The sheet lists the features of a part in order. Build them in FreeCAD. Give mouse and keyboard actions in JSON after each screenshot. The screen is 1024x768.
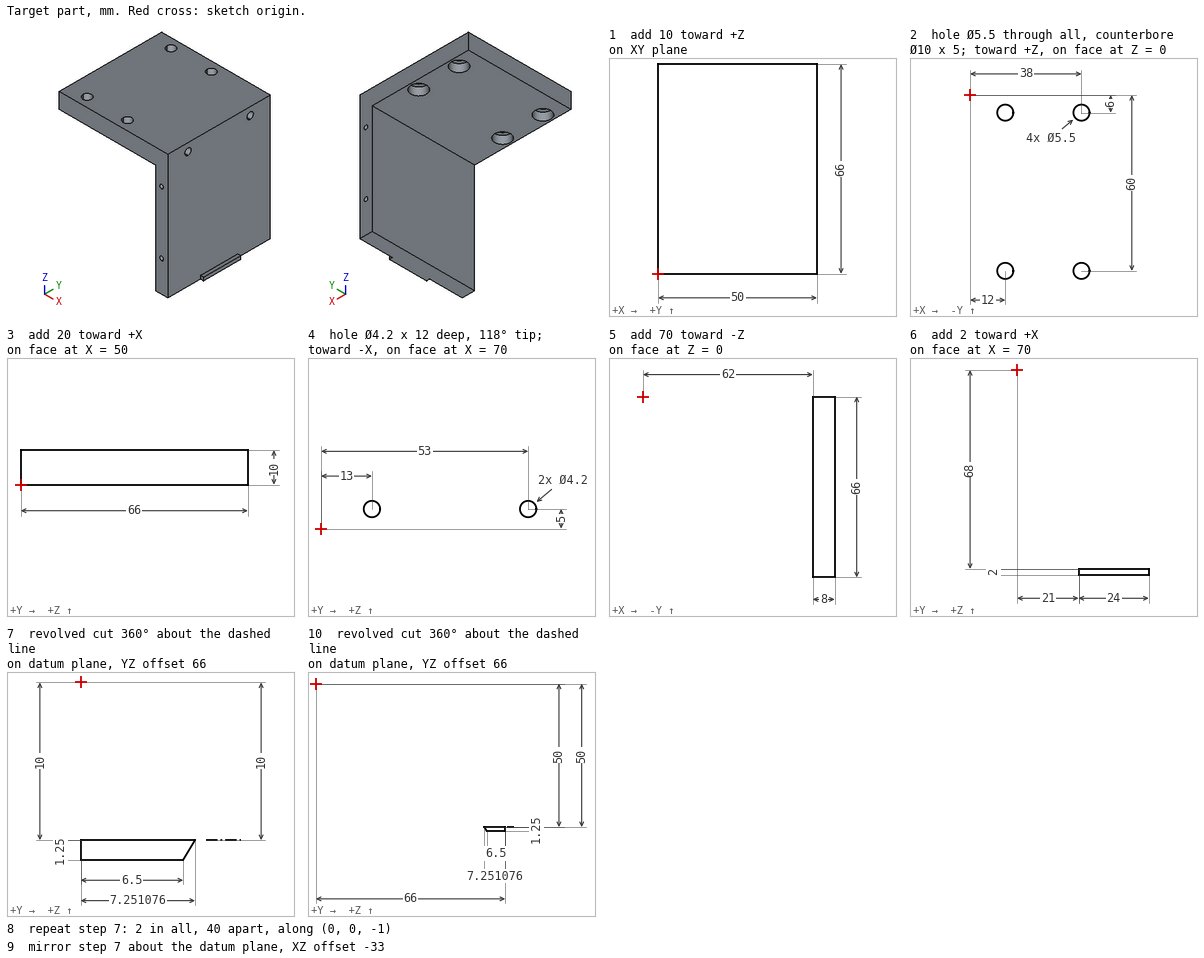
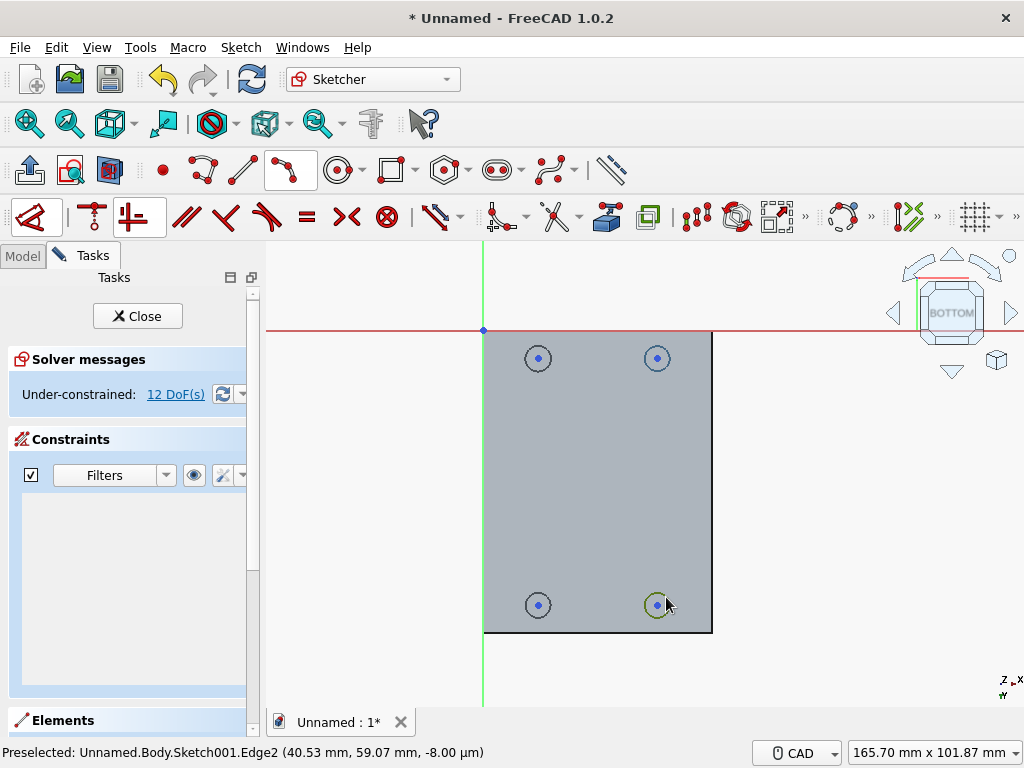
{"action": "left_click", "coordinate": [547, 597]}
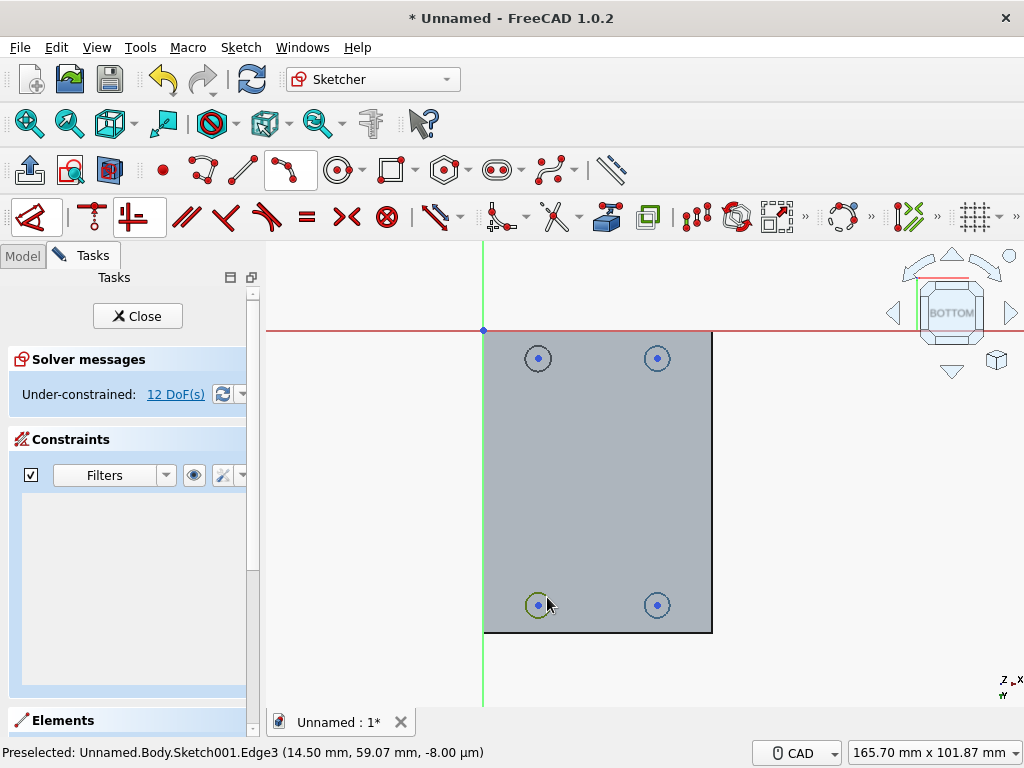
{"action": "left_click", "coordinate": [547, 350]}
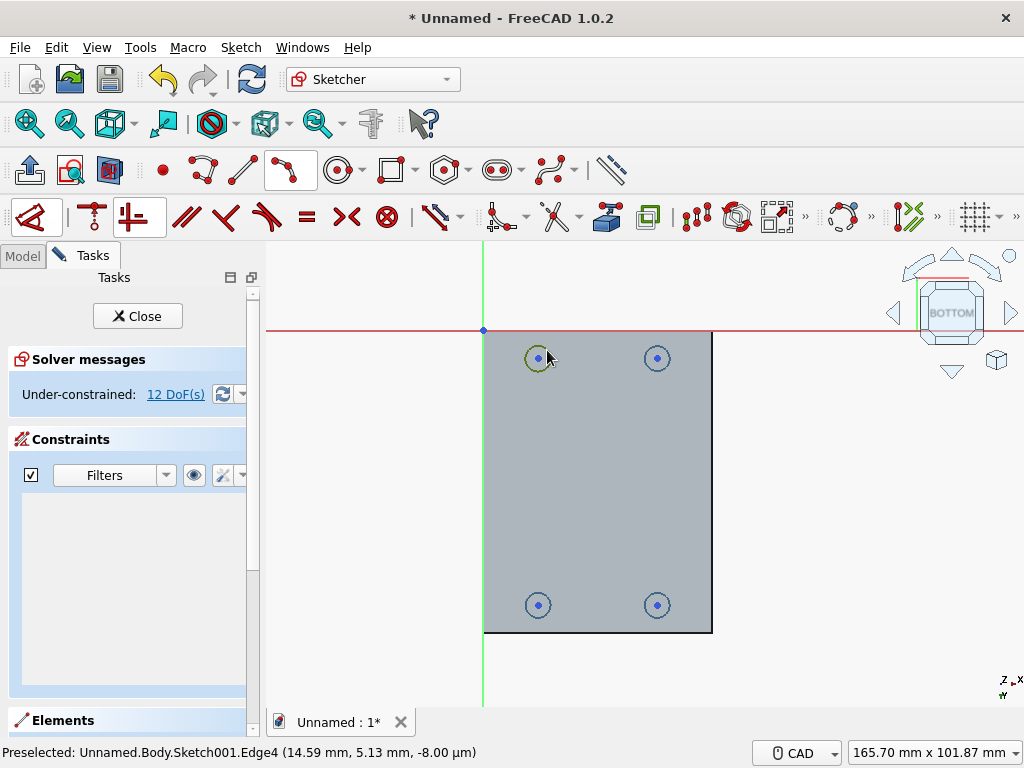
{"action": "left_click", "coordinate": [308, 218]}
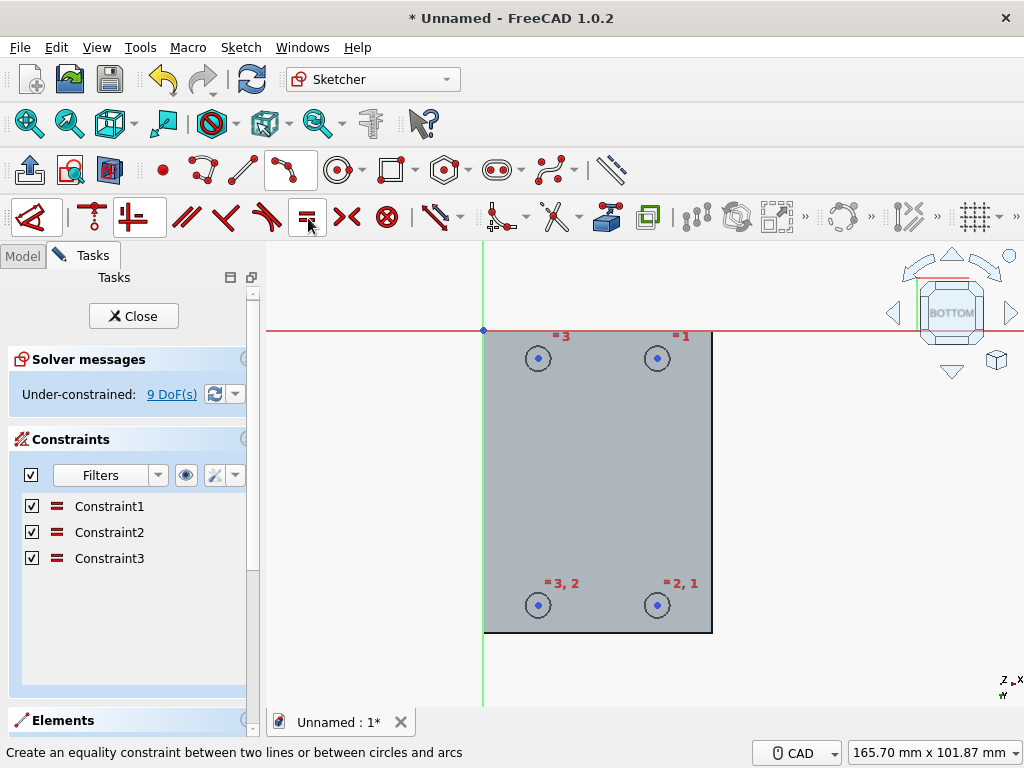
{"action": "left_click", "coordinate": [657, 359]}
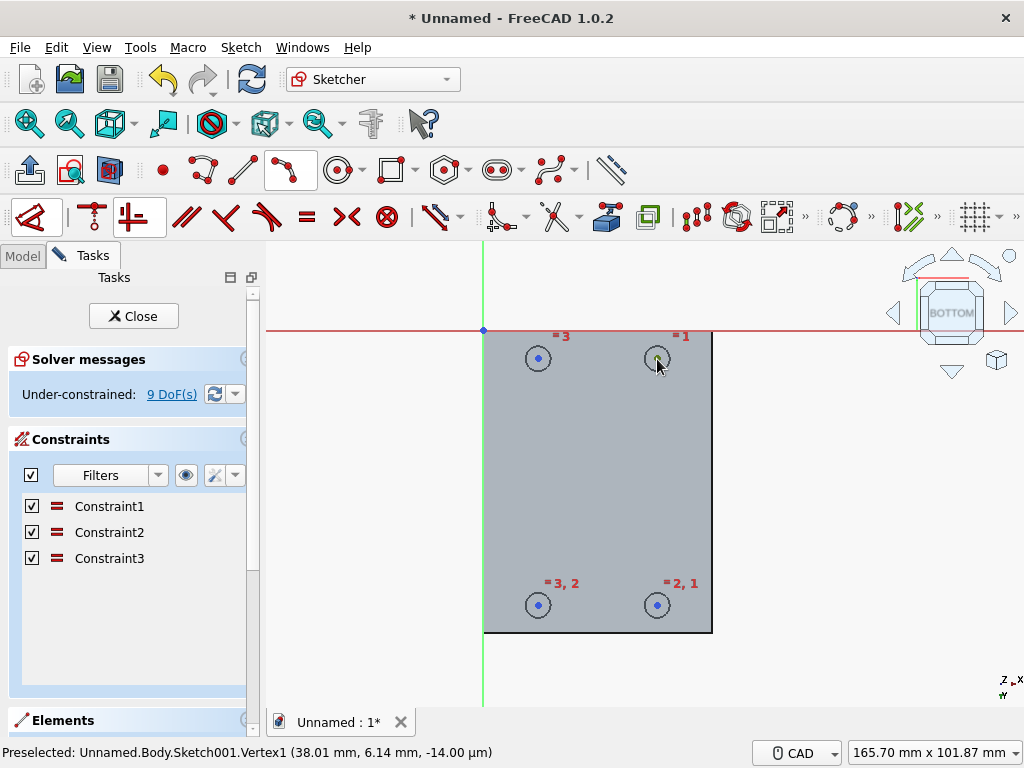
{"action": "left_click", "coordinate": [657, 605]}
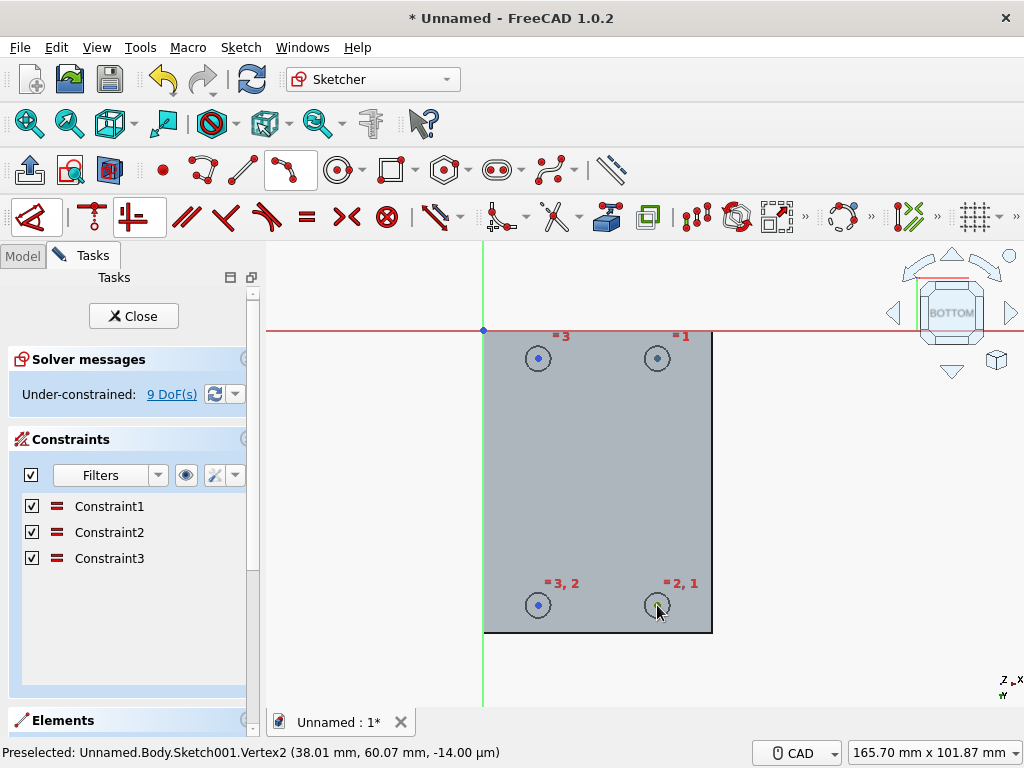
{"action": "key", "text": "v"}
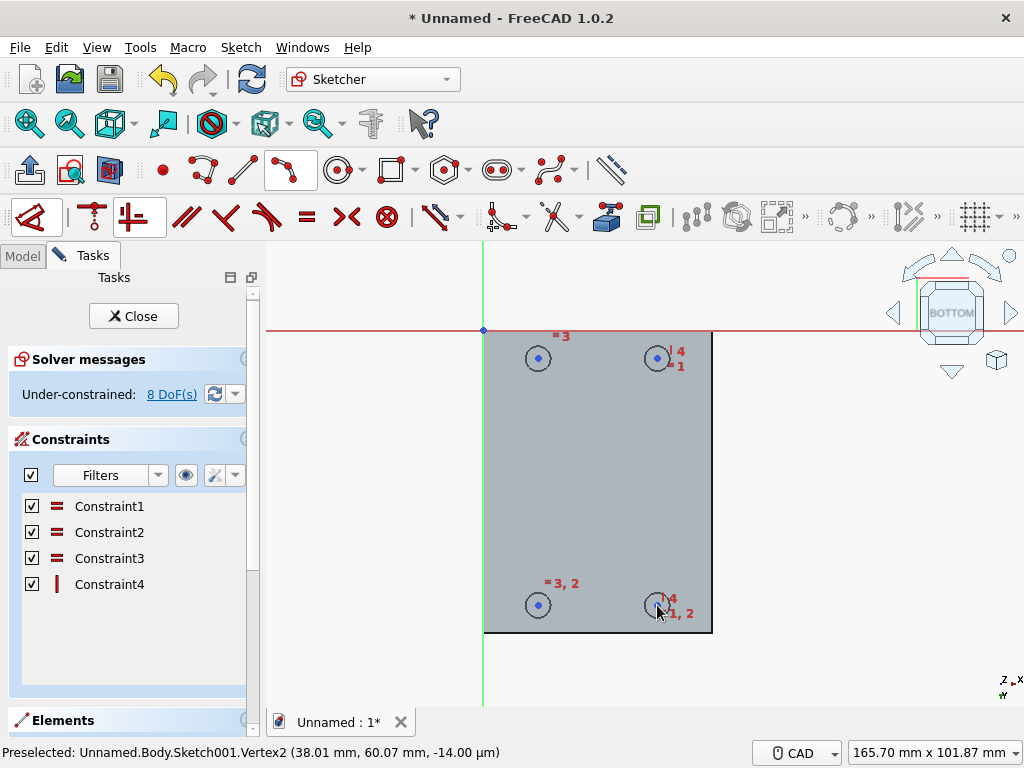
{"action": "left_click", "coordinate": [657, 605]}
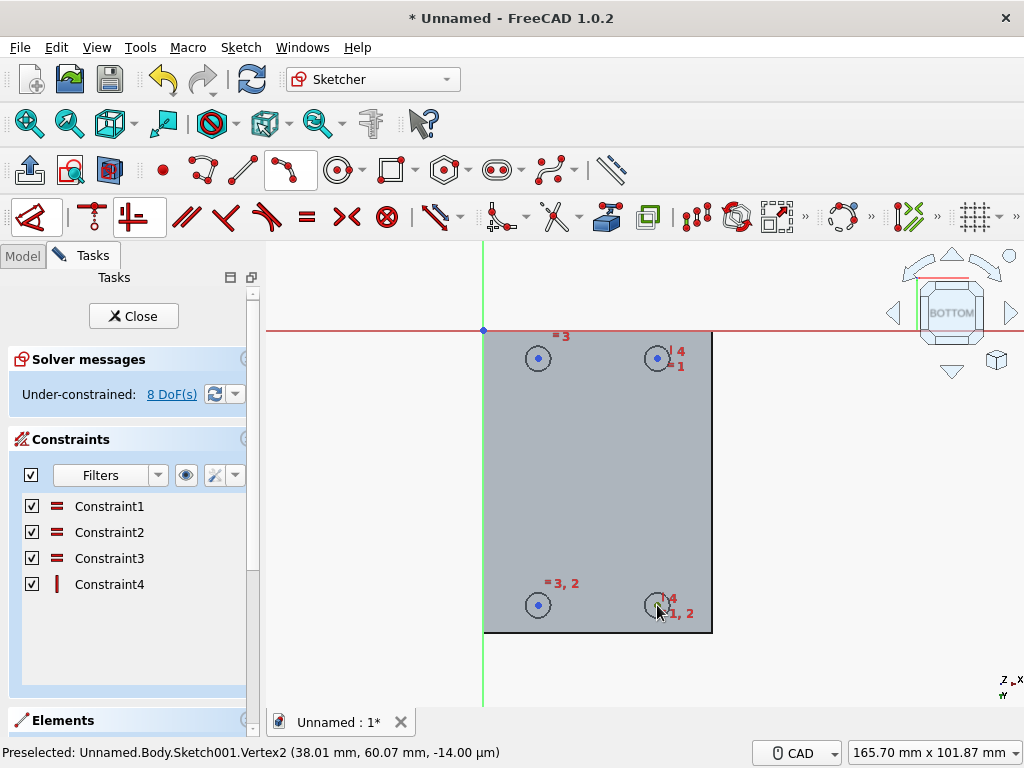
{"action": "left_click", "coordinate": [538, 605]}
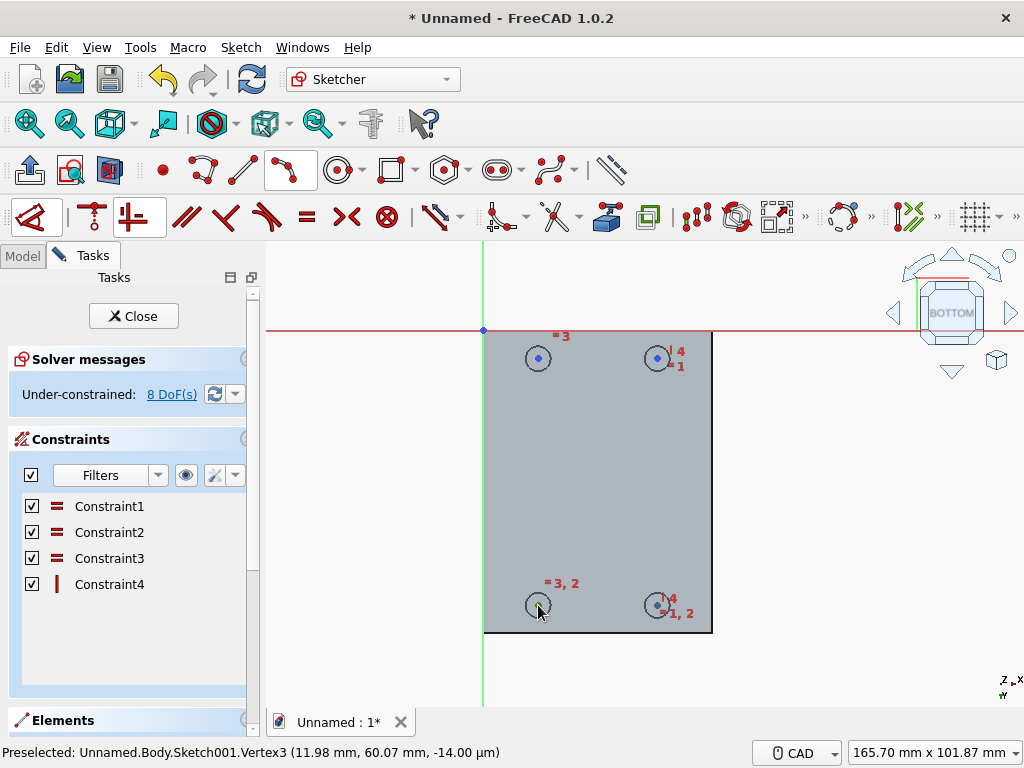
{"action": "key", "text": "h"}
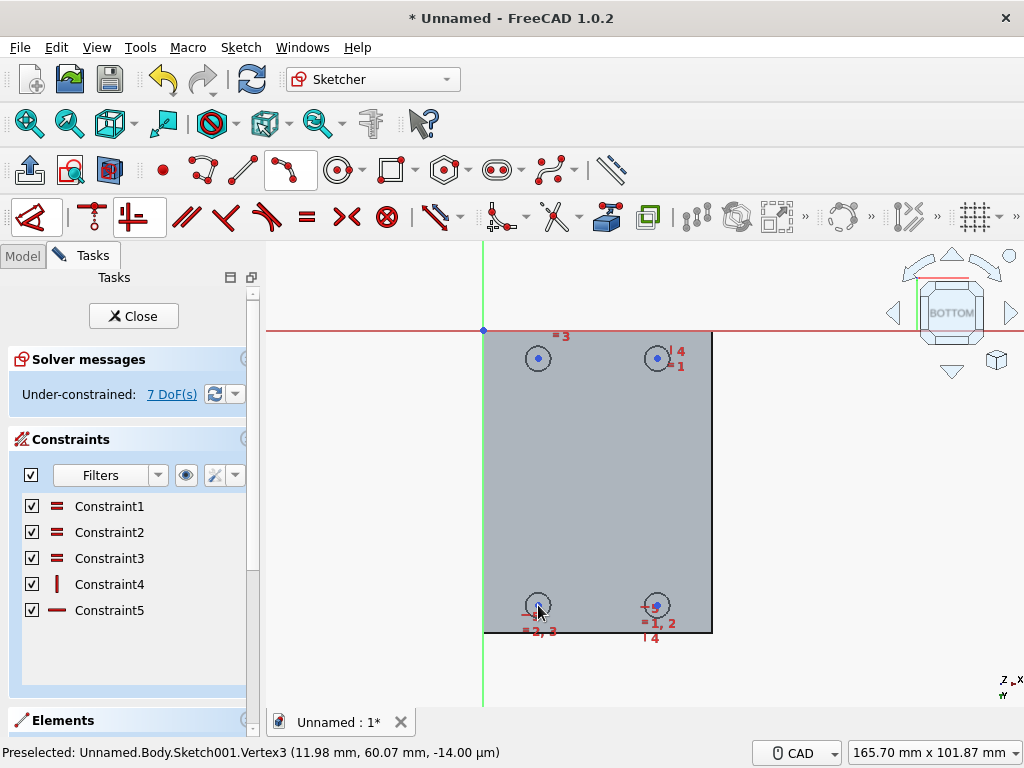
{"action": "left_click", "coordinate": [538, 605]}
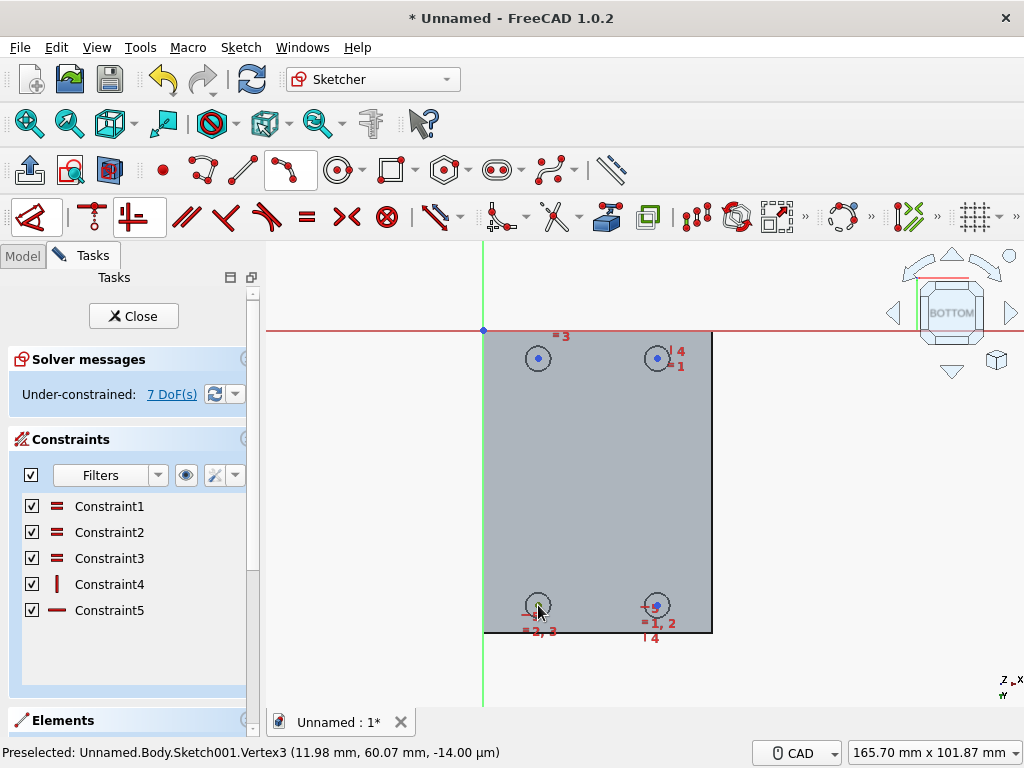
{"action": "left_click", "coordinate": [538, 359]}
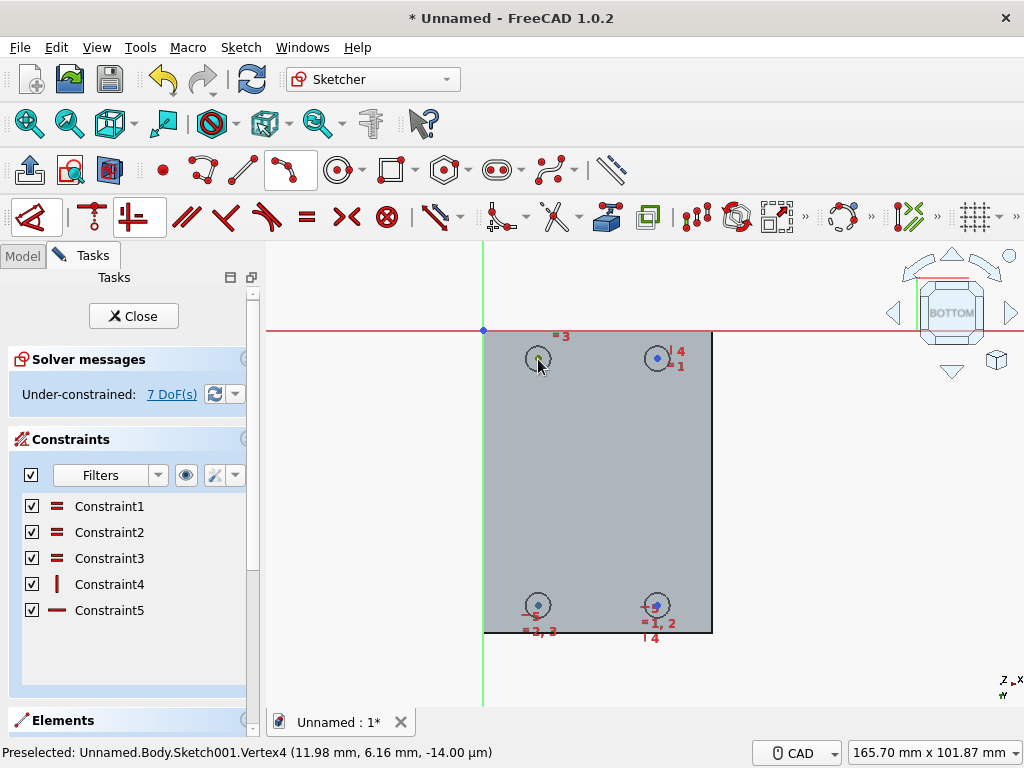
{"action": "key", "text": "v"}